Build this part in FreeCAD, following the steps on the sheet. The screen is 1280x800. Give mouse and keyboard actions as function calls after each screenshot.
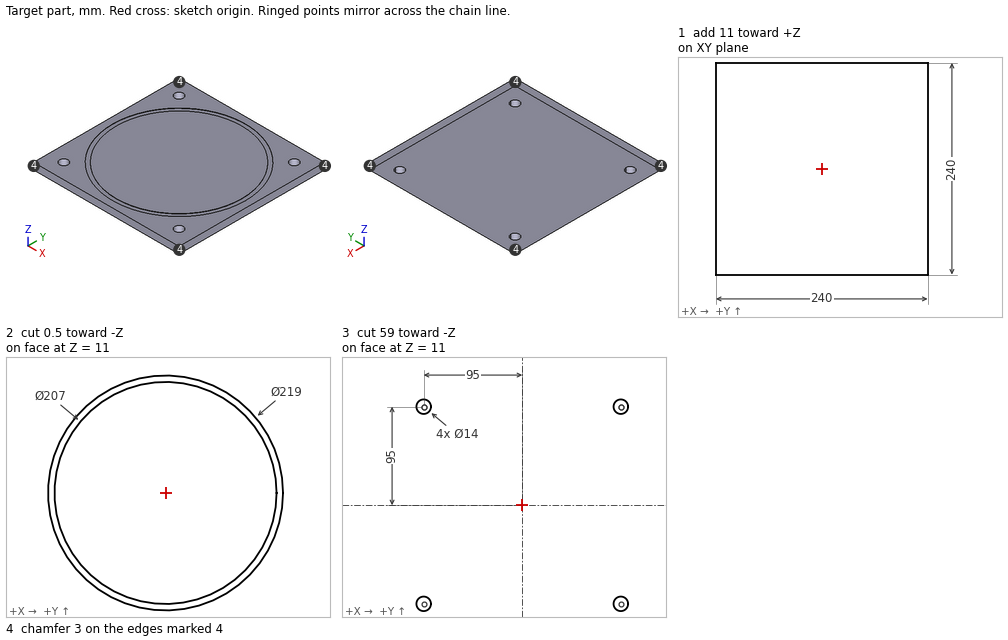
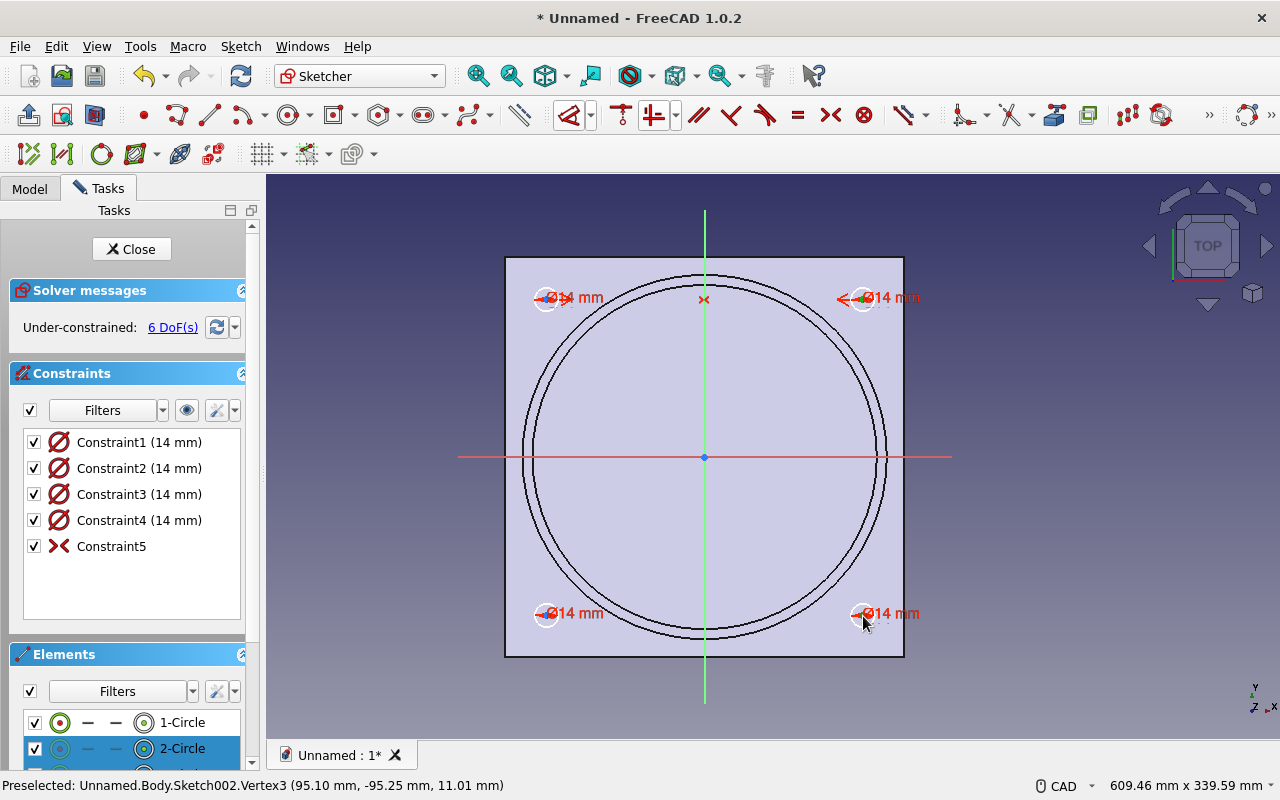
click(470, 457)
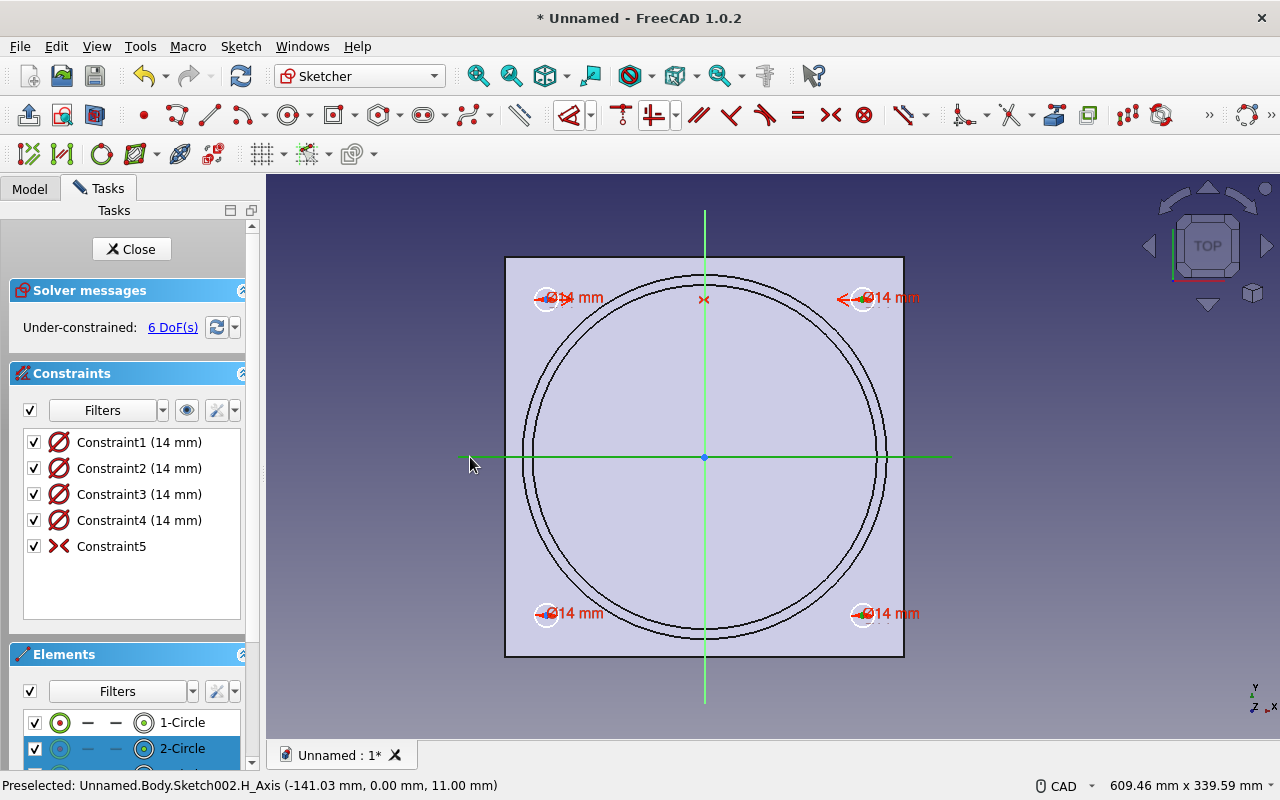
click(831, 116)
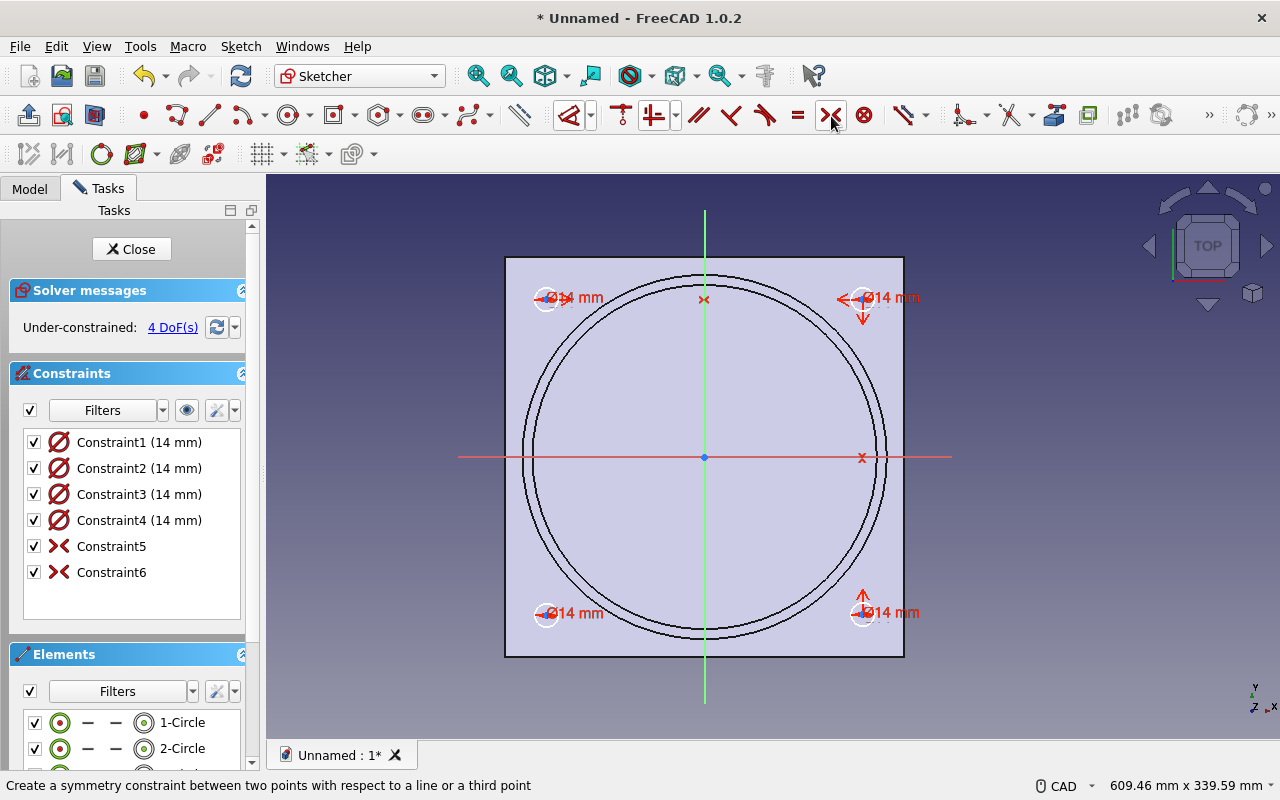
click(546, 300)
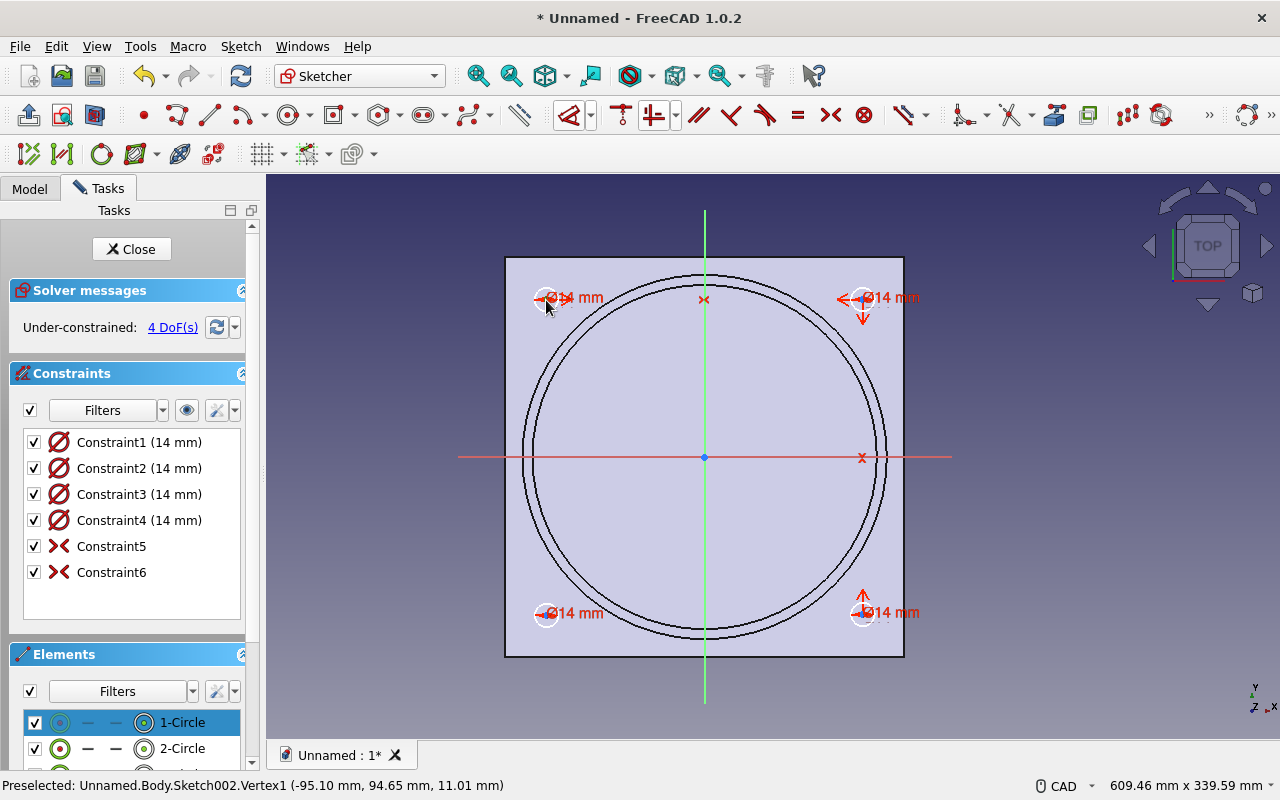
click(547, 615)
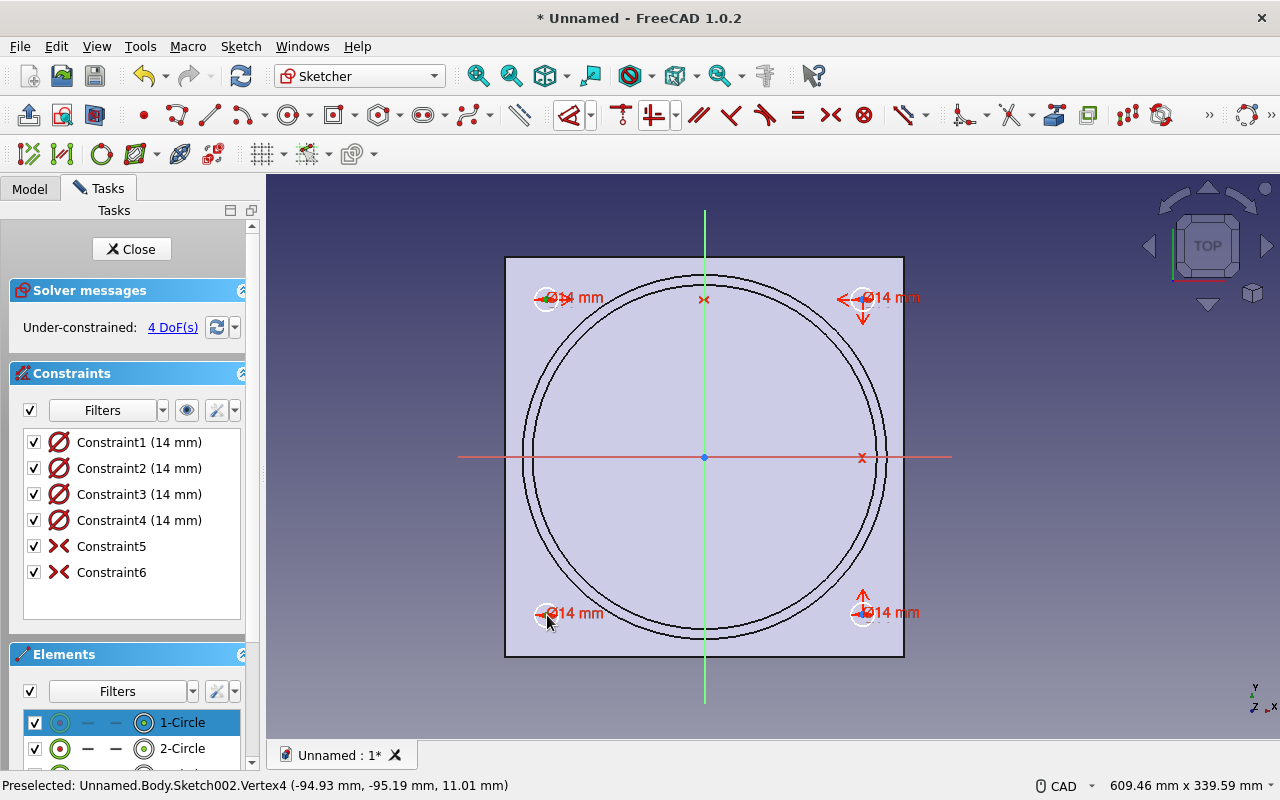
click(470, 457)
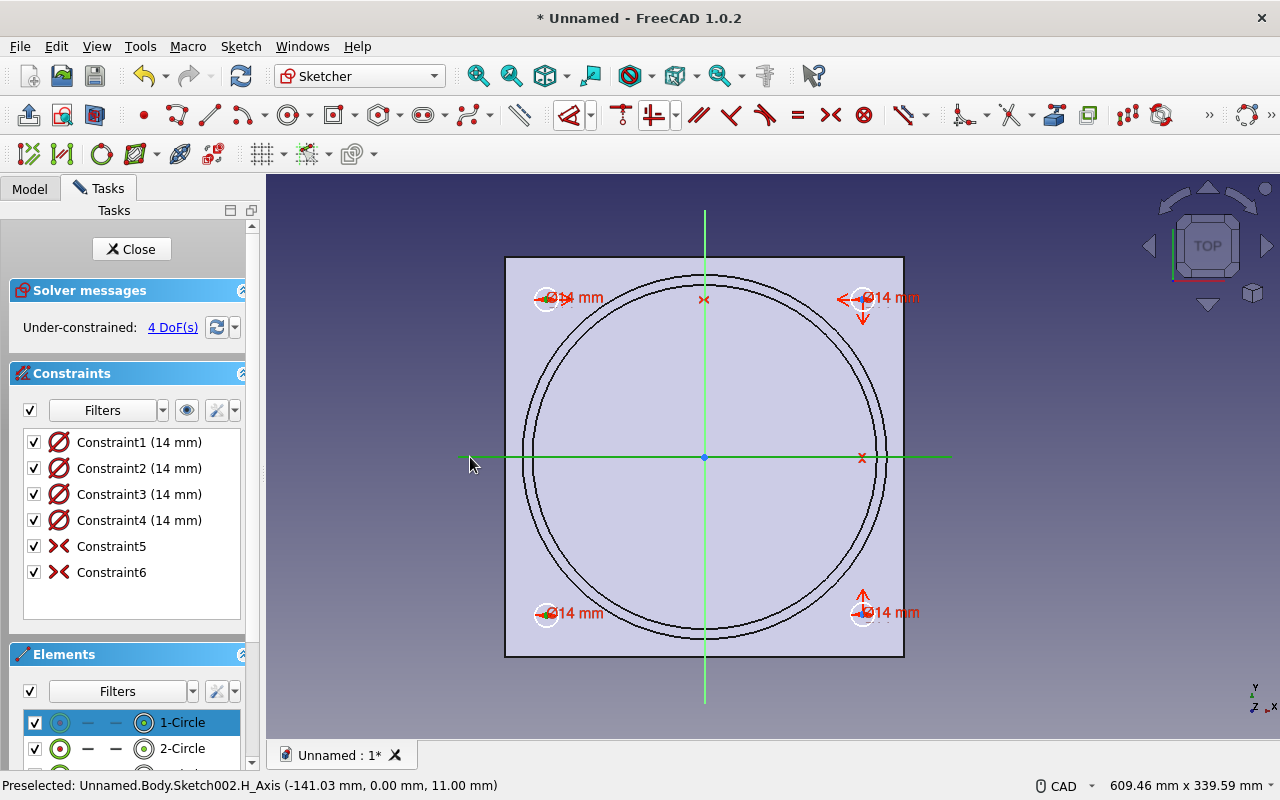
click(831, 116)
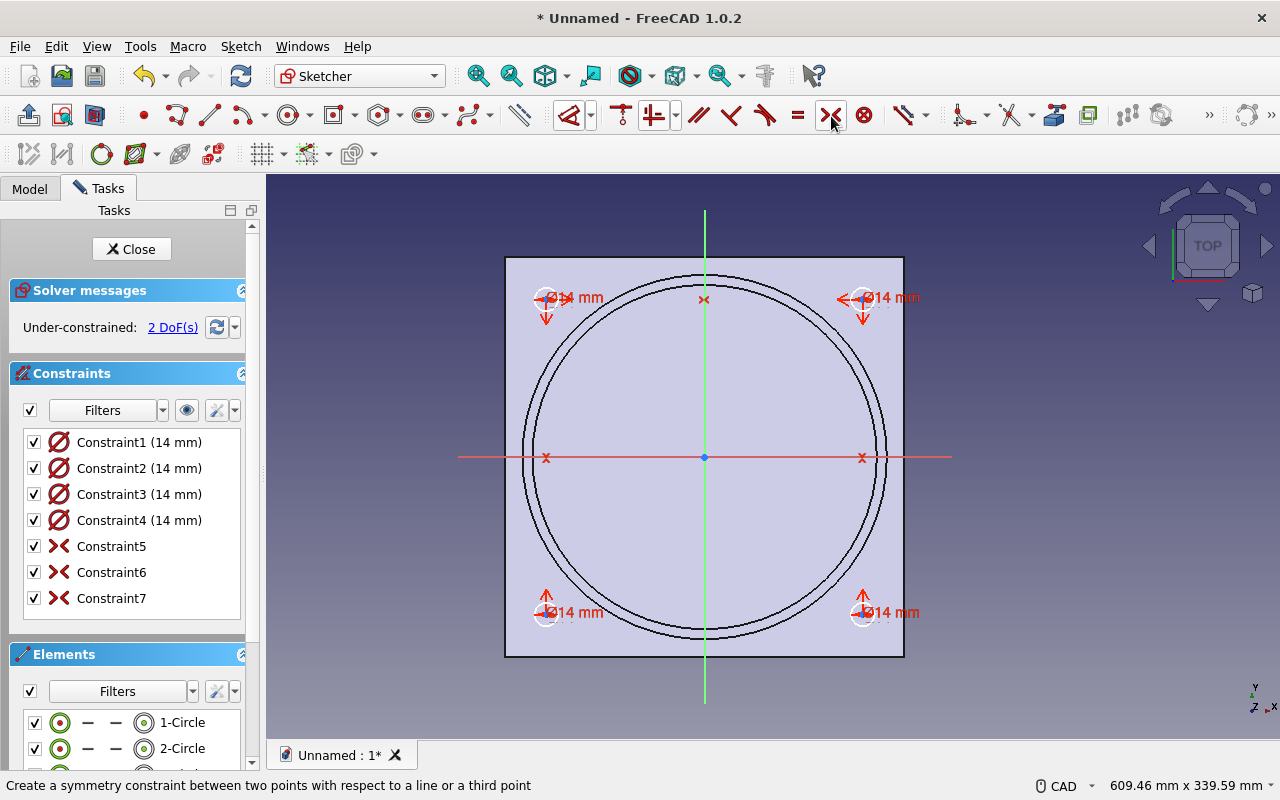
click(546, 300)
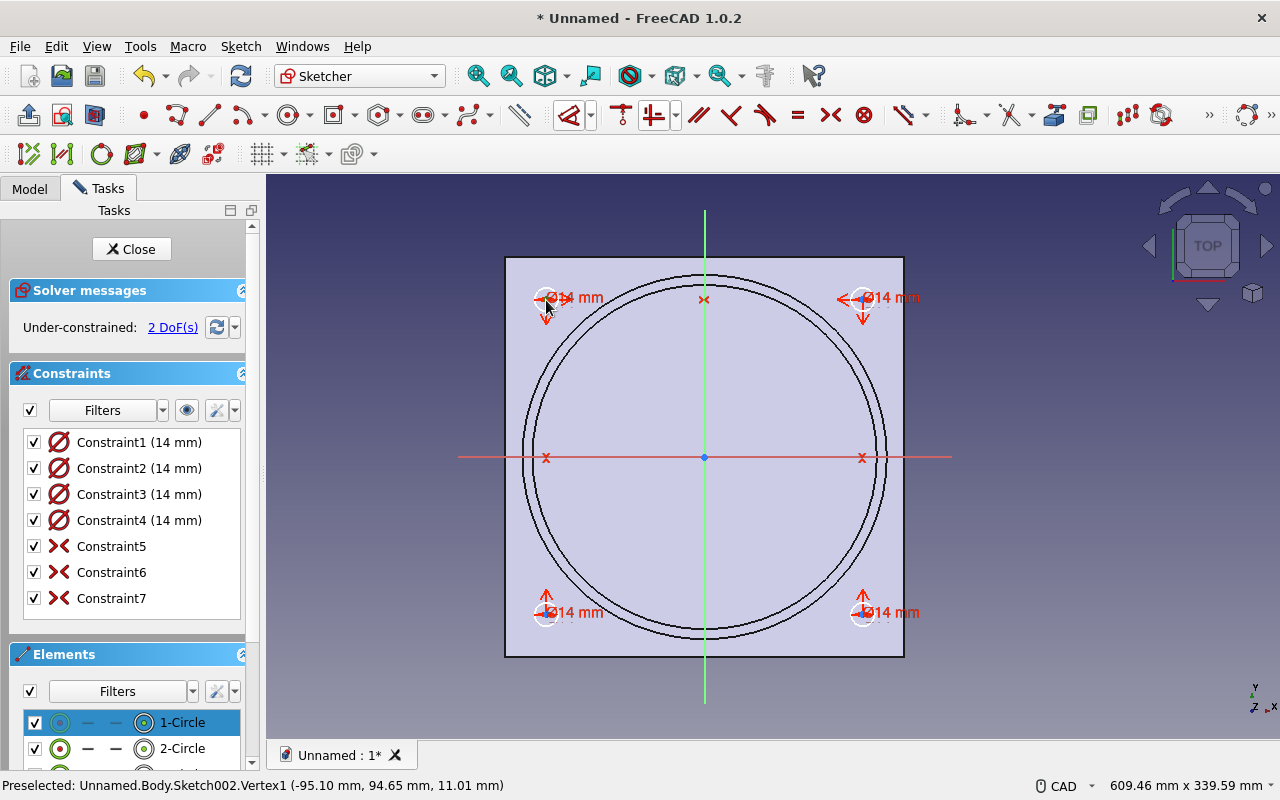
key(l)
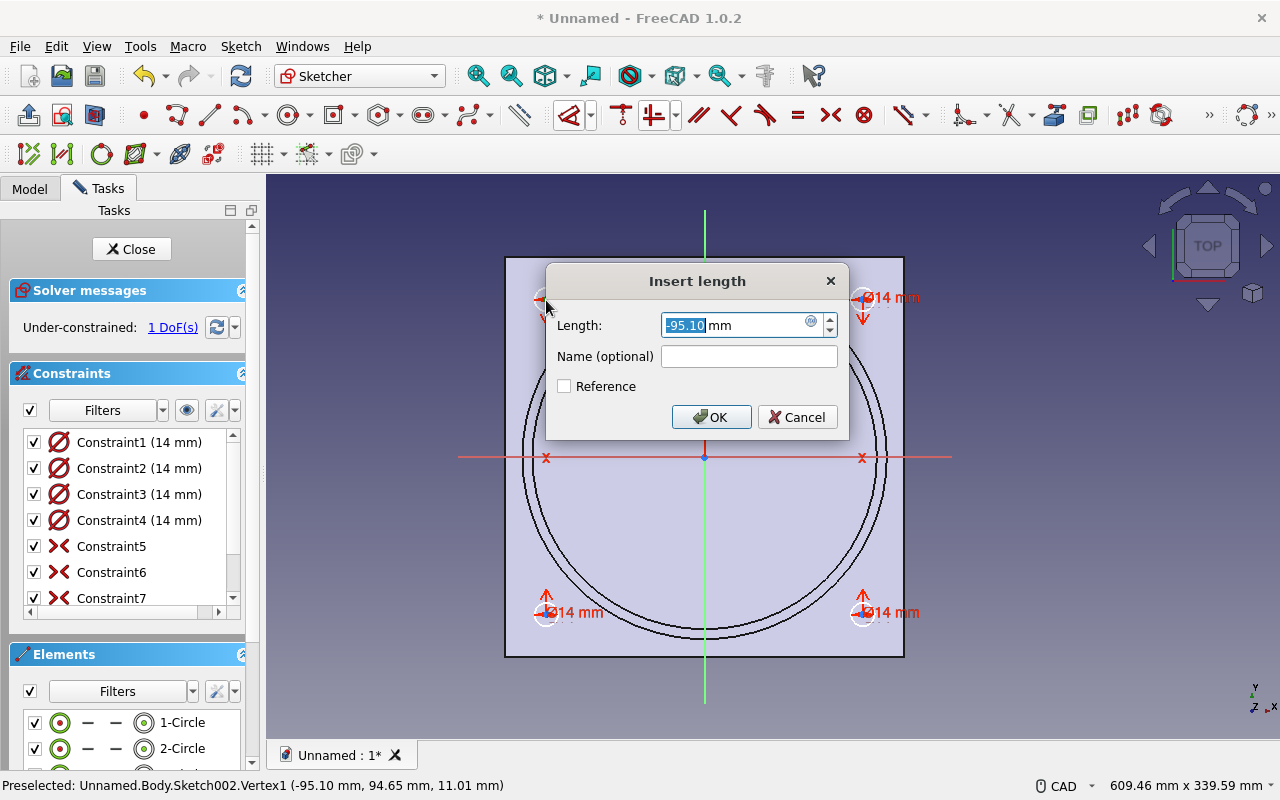
text(-95)
key(Return)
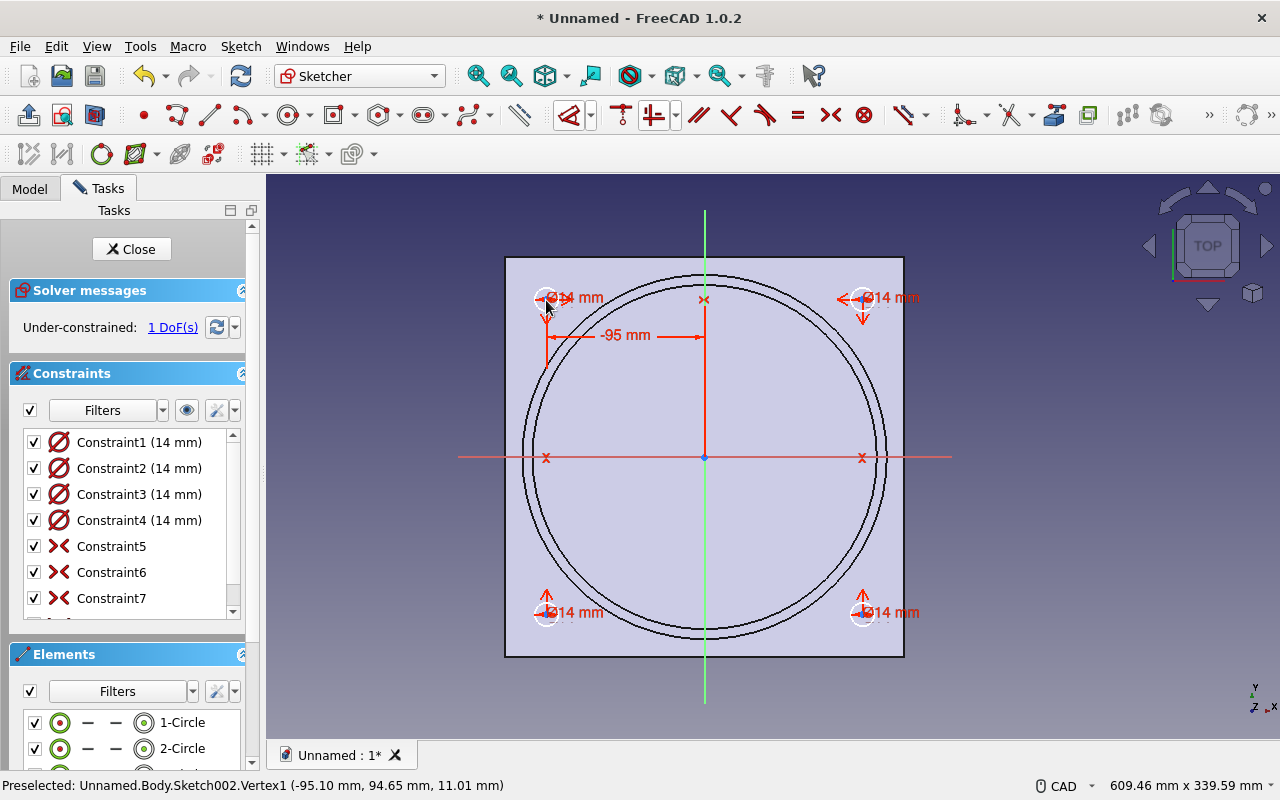
click(547, 300)